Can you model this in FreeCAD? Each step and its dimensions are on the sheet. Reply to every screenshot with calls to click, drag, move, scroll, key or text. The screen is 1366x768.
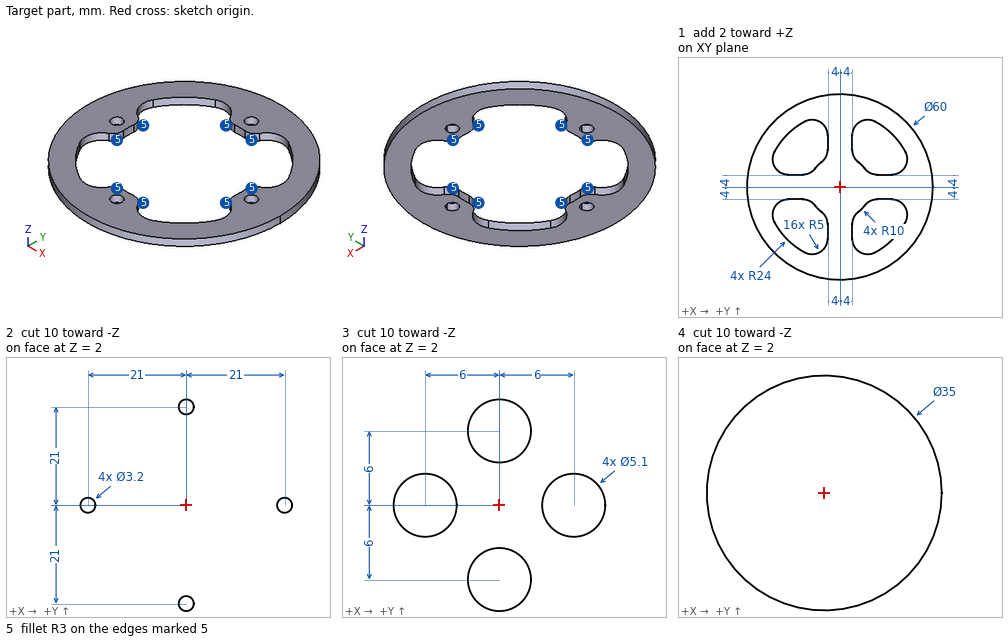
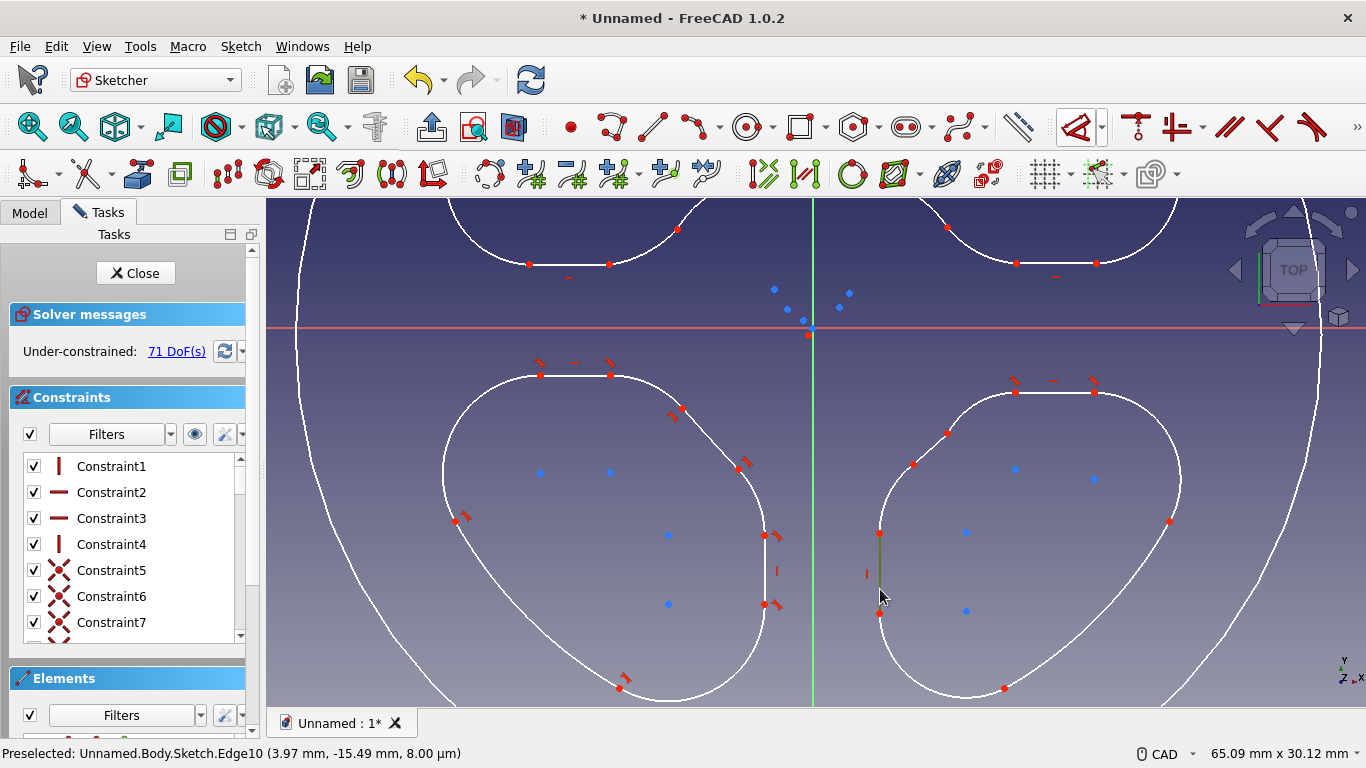
click(896, 662)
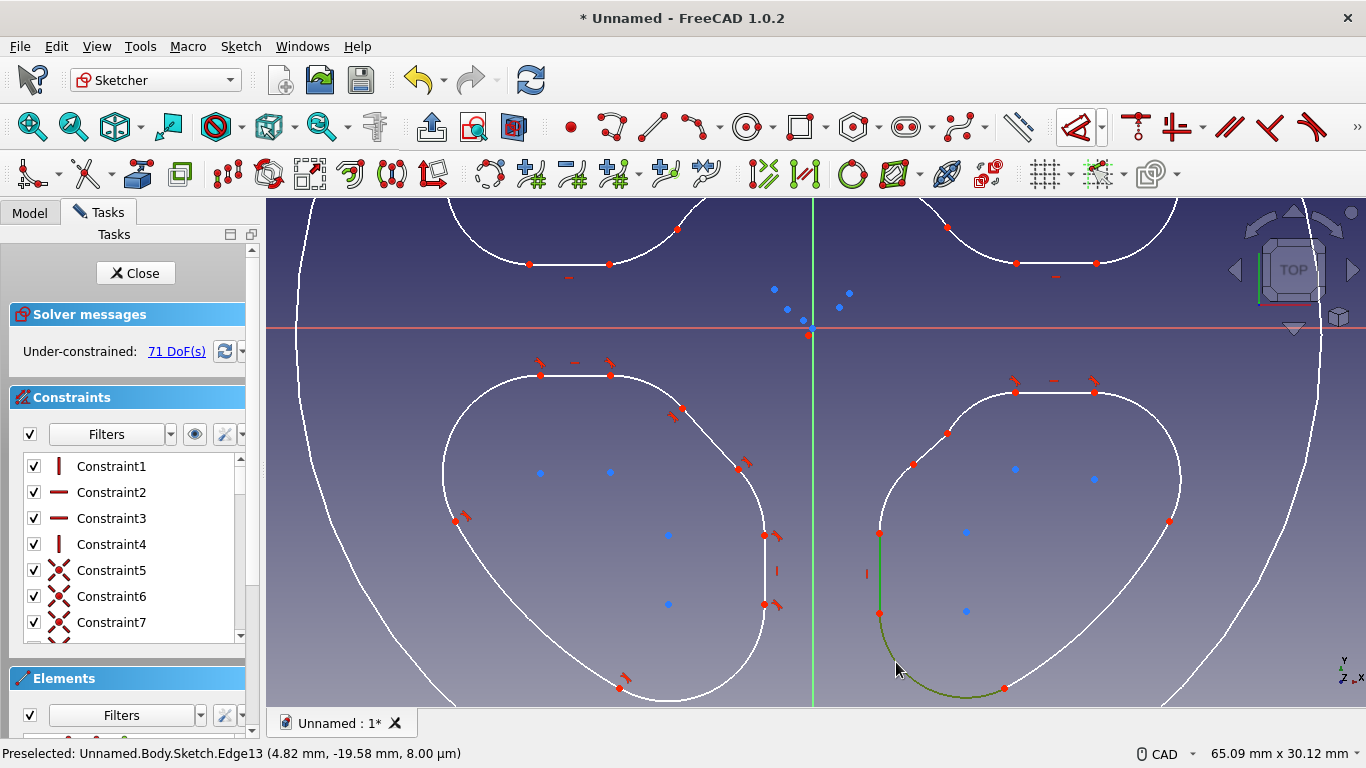
key(t)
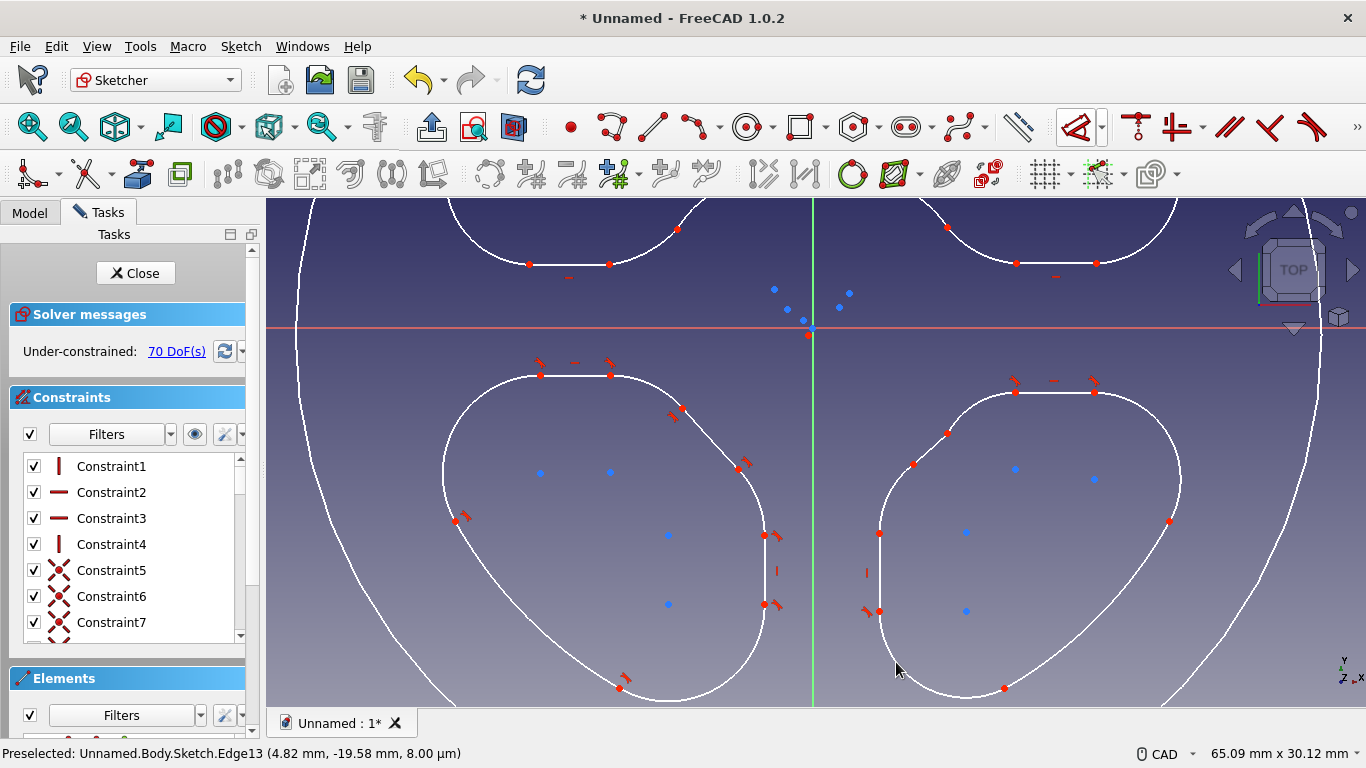
click(880, 588)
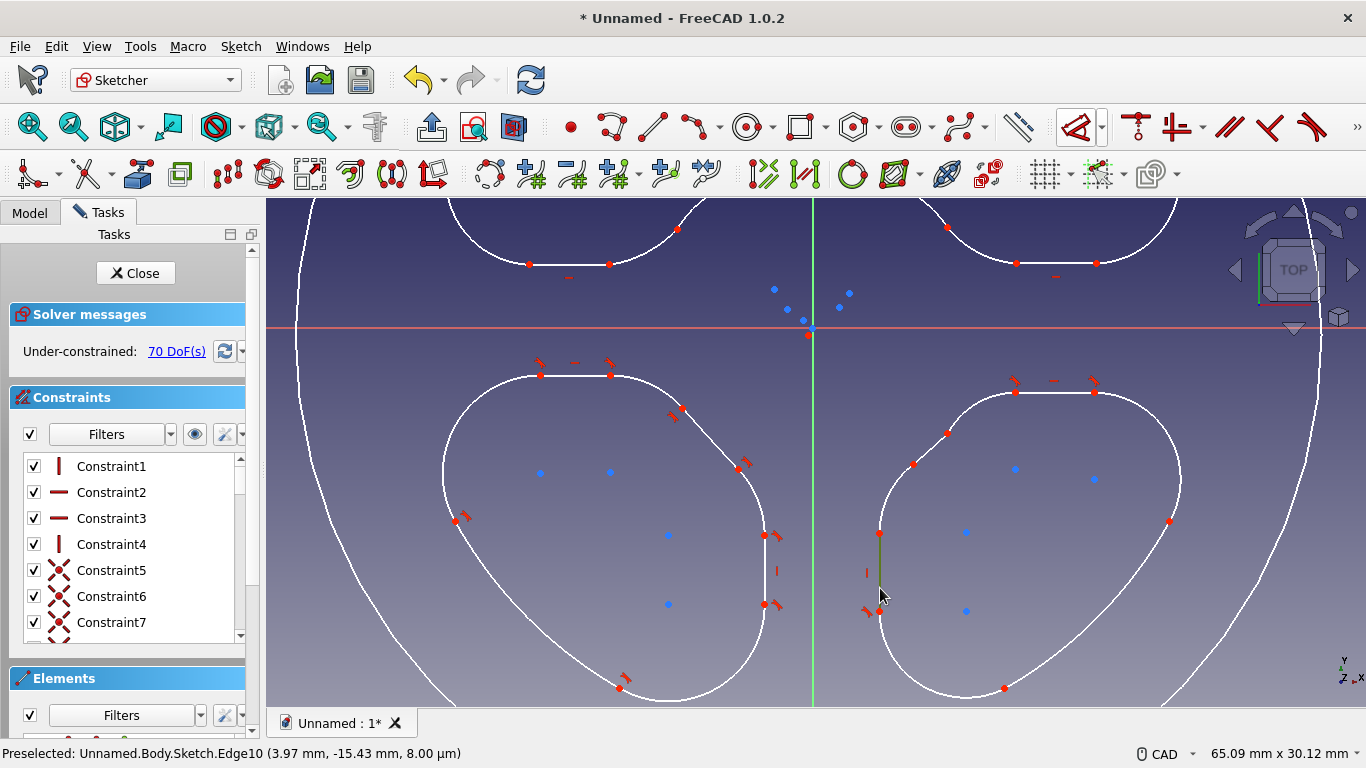
click(897, 481)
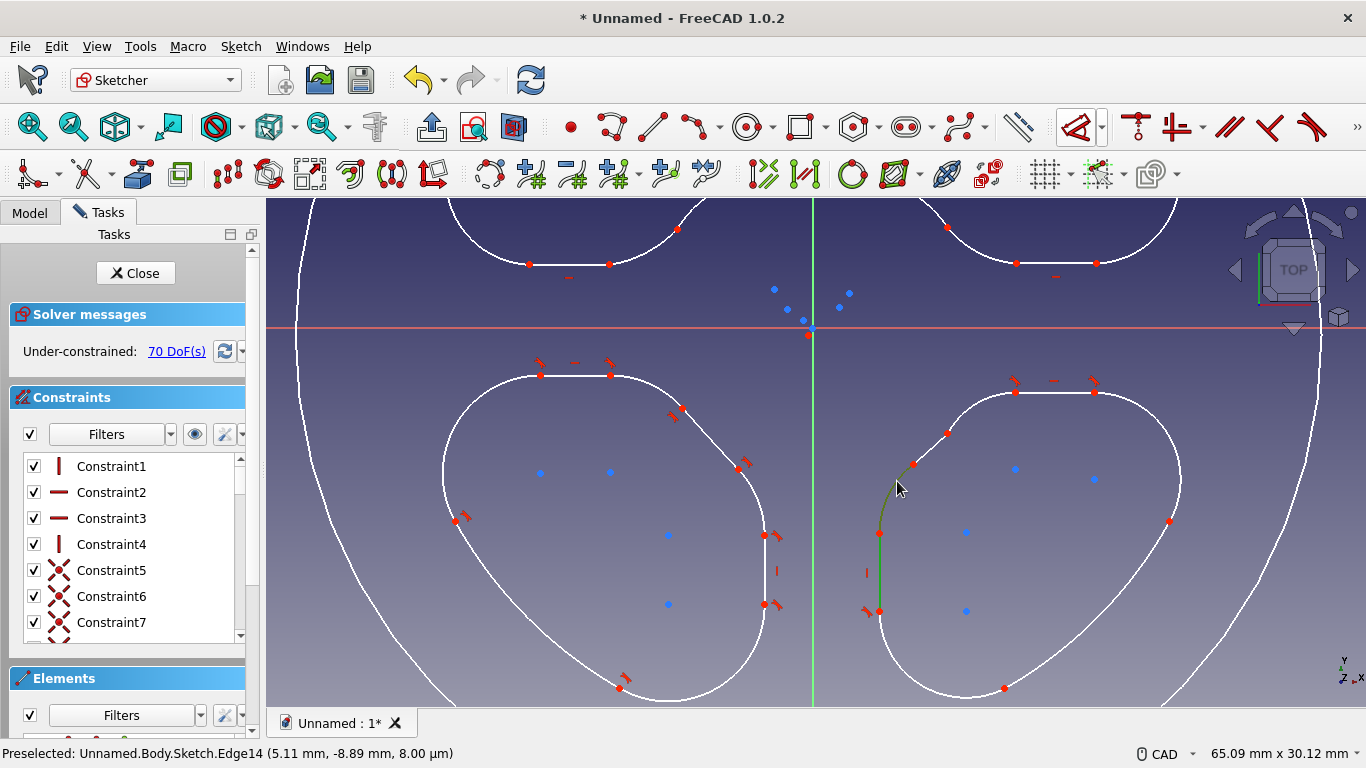
key(t)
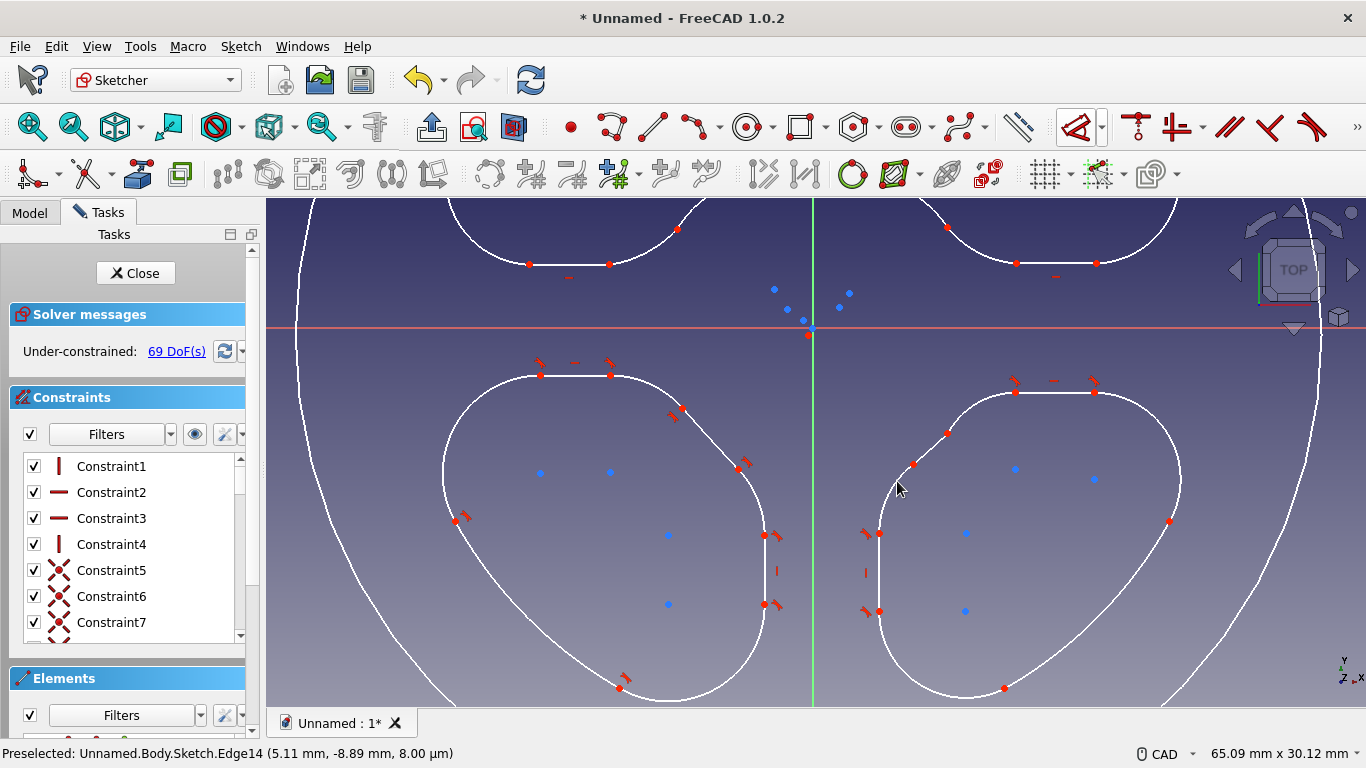
click(1180, 470)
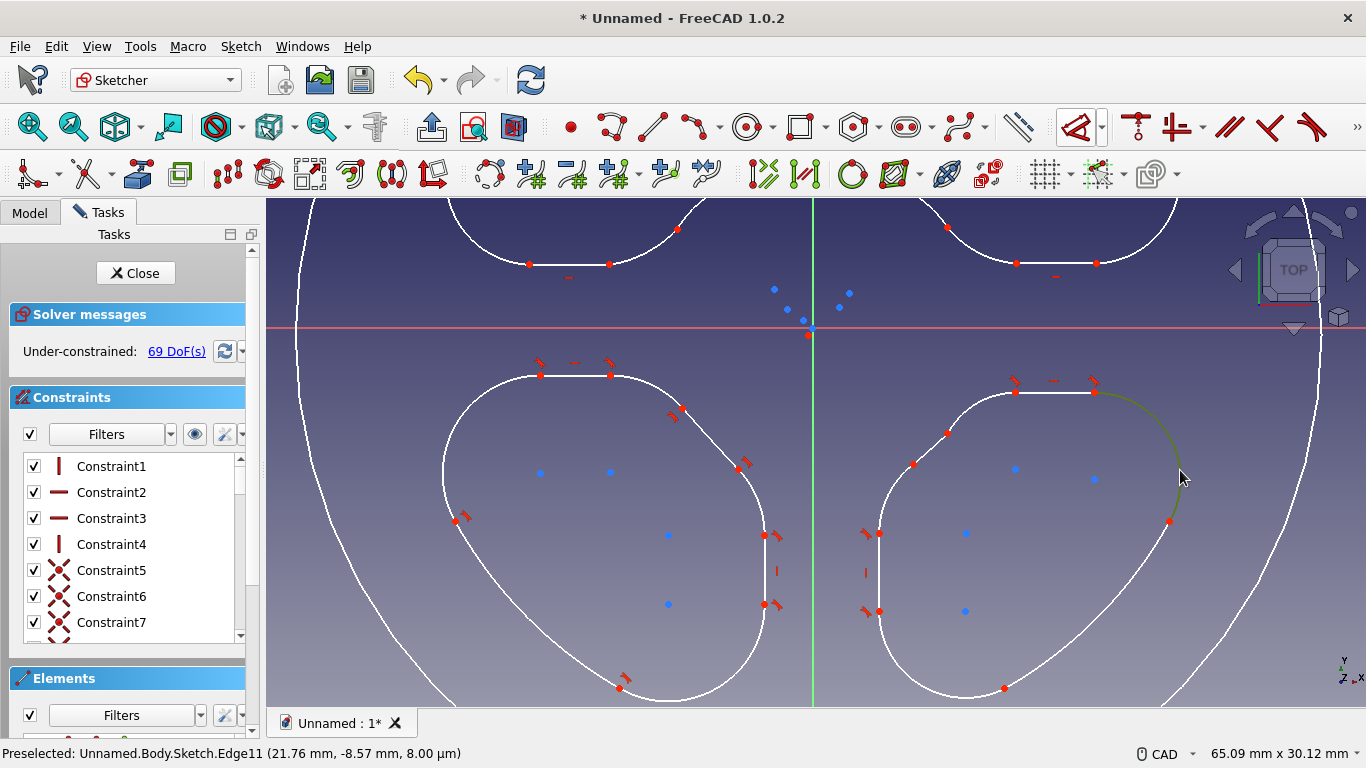
click(1063, 648)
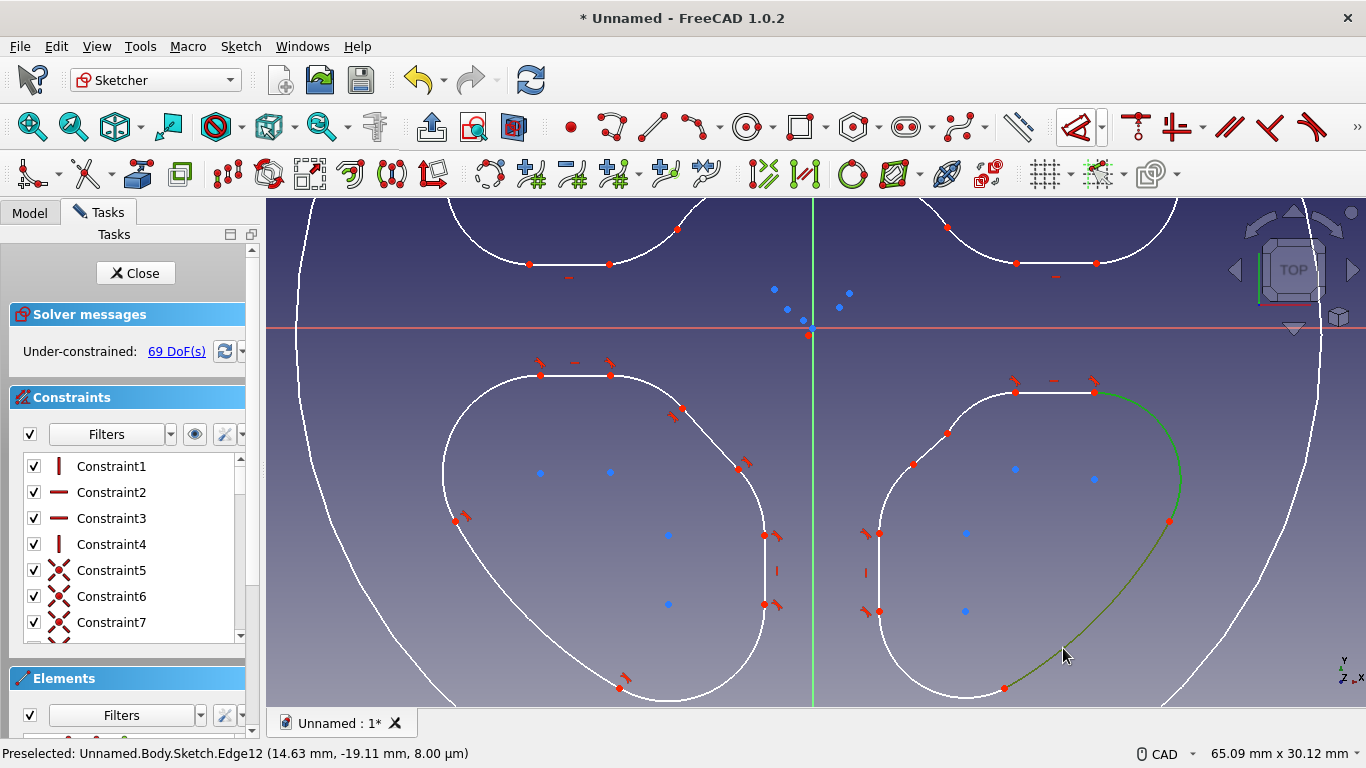
key(t)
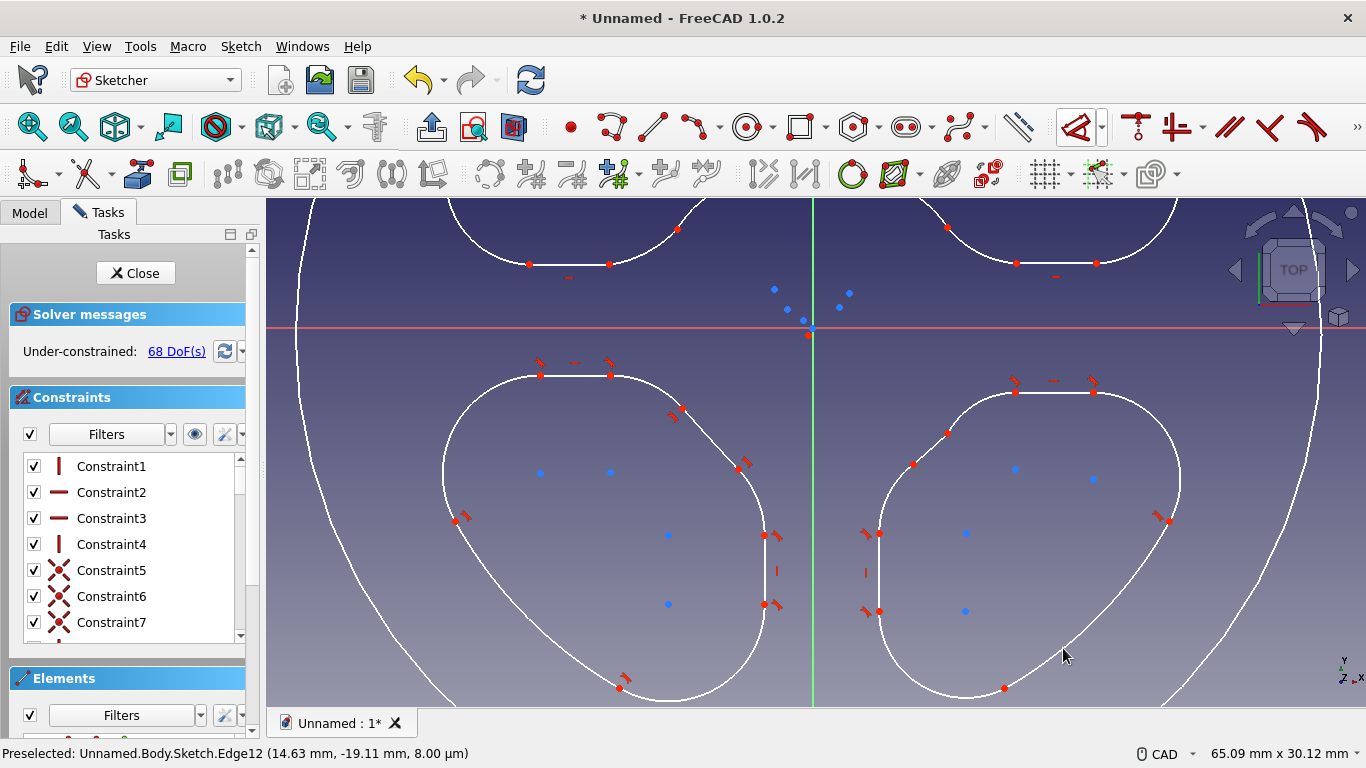
click(1063, 648)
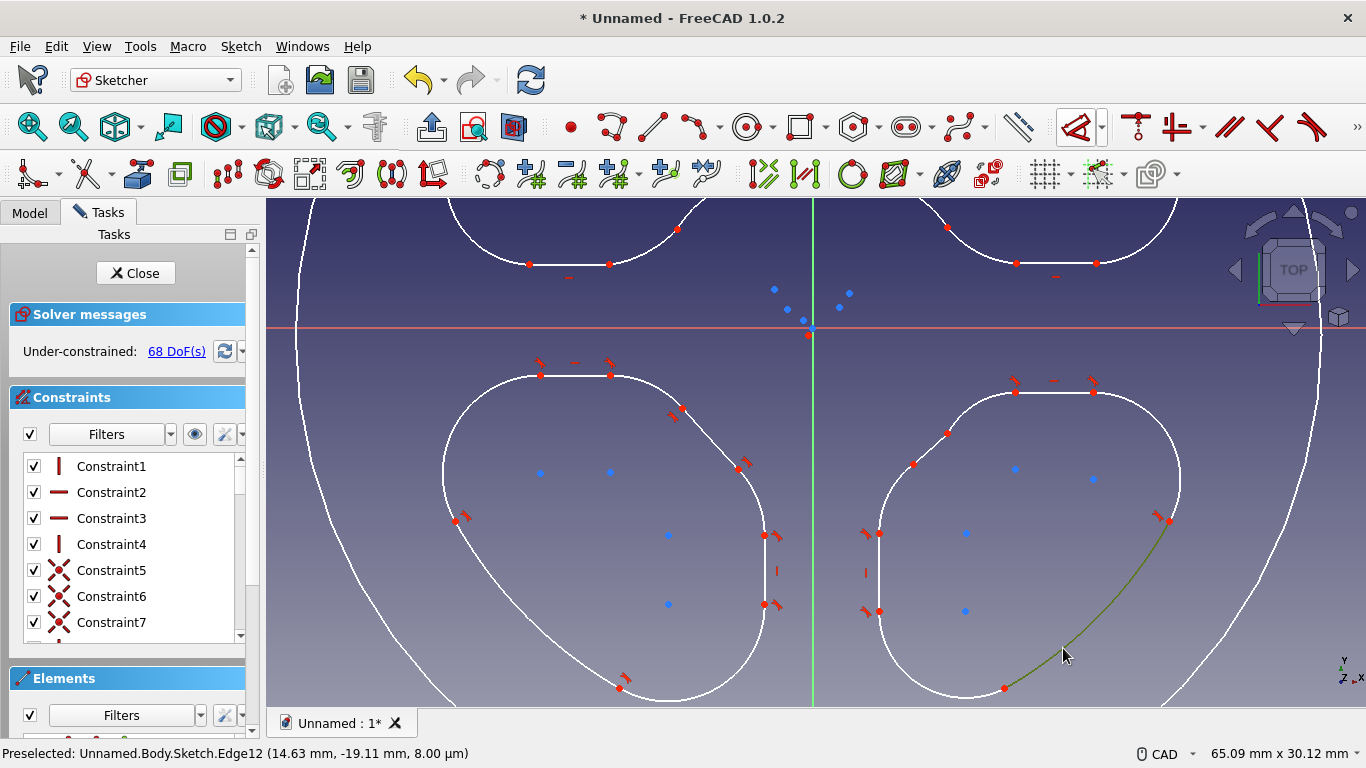
click(895, 661)